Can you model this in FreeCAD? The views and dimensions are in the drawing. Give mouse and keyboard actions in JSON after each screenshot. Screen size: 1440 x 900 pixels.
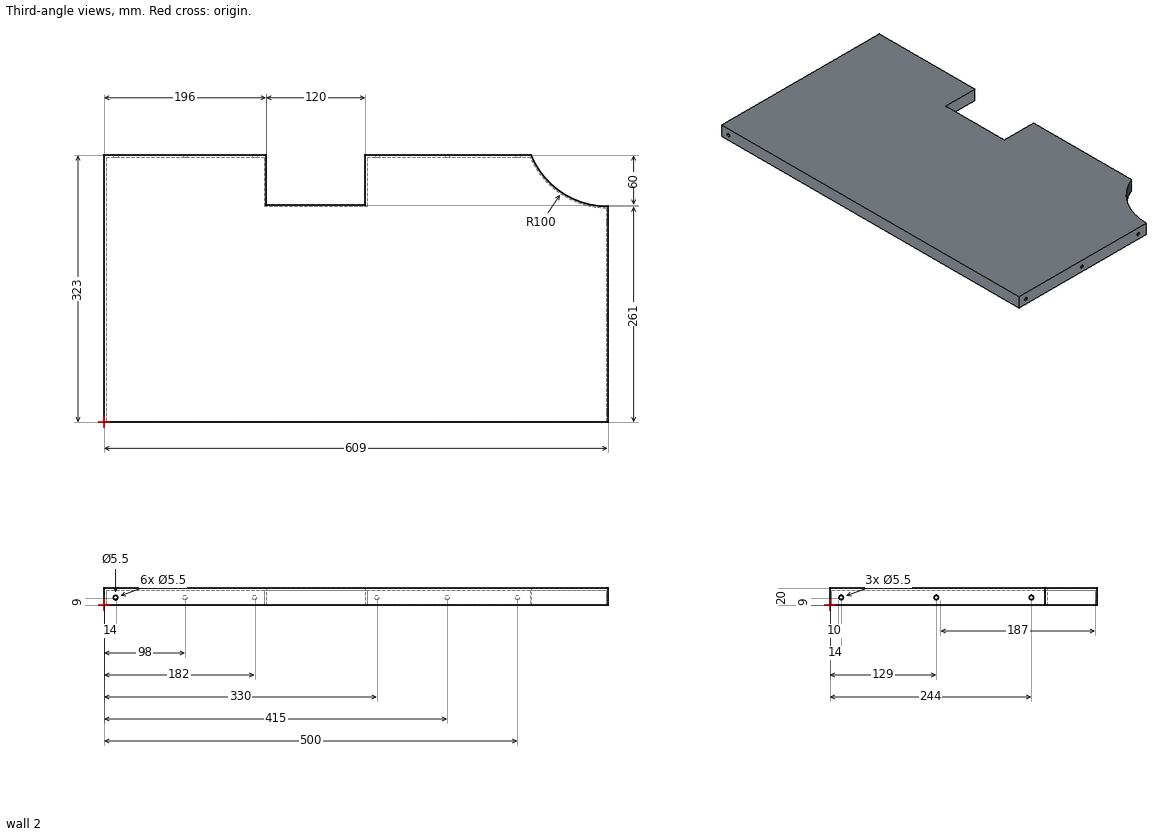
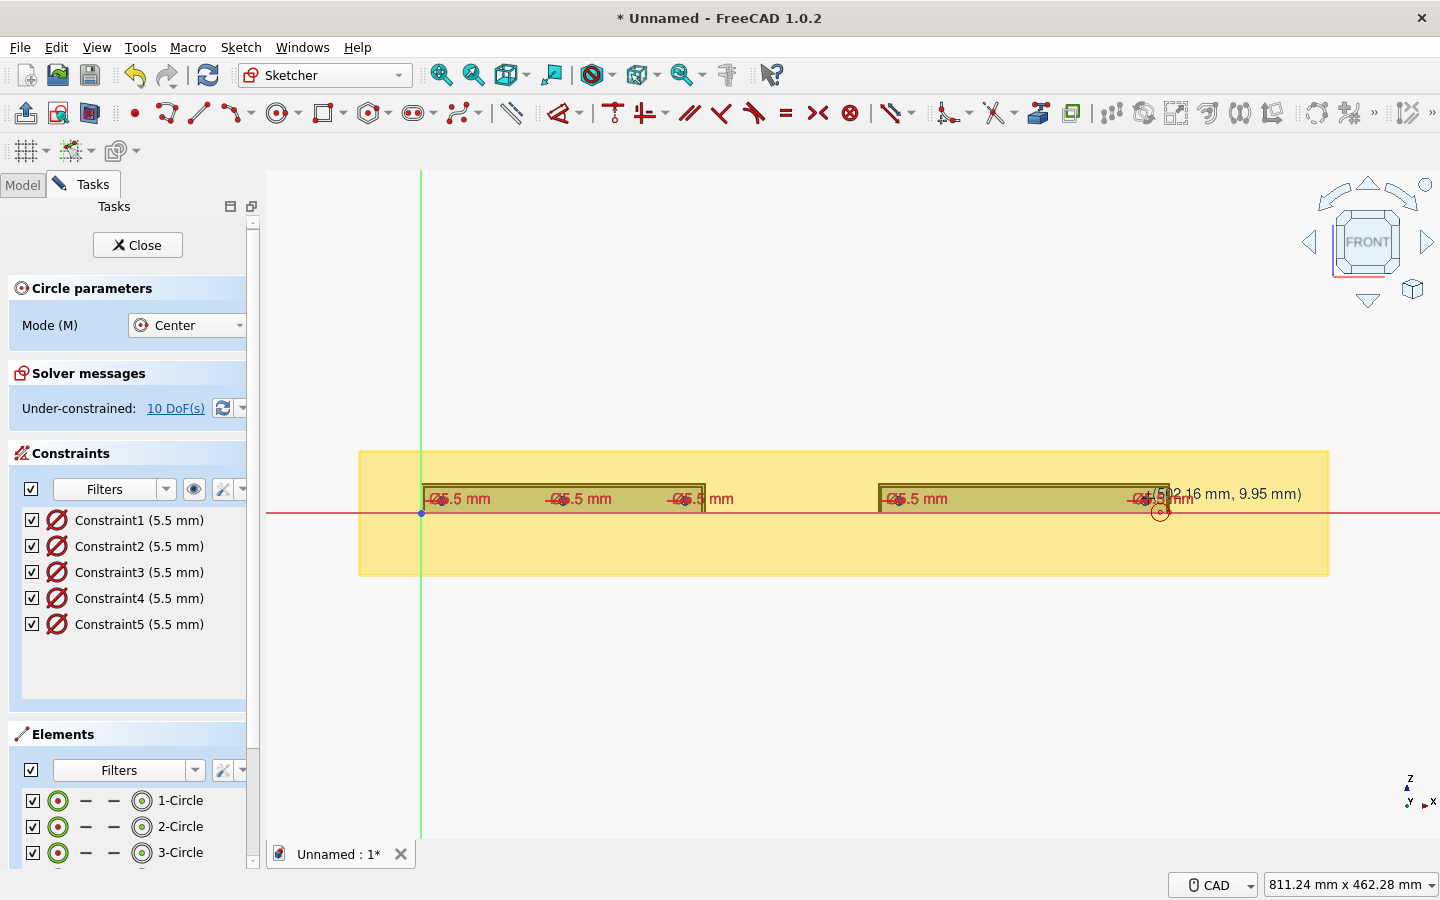
{"action": "scroll", "coordinate": [1022, 500], "scroll_direction": "up", "scroll_amount": 9}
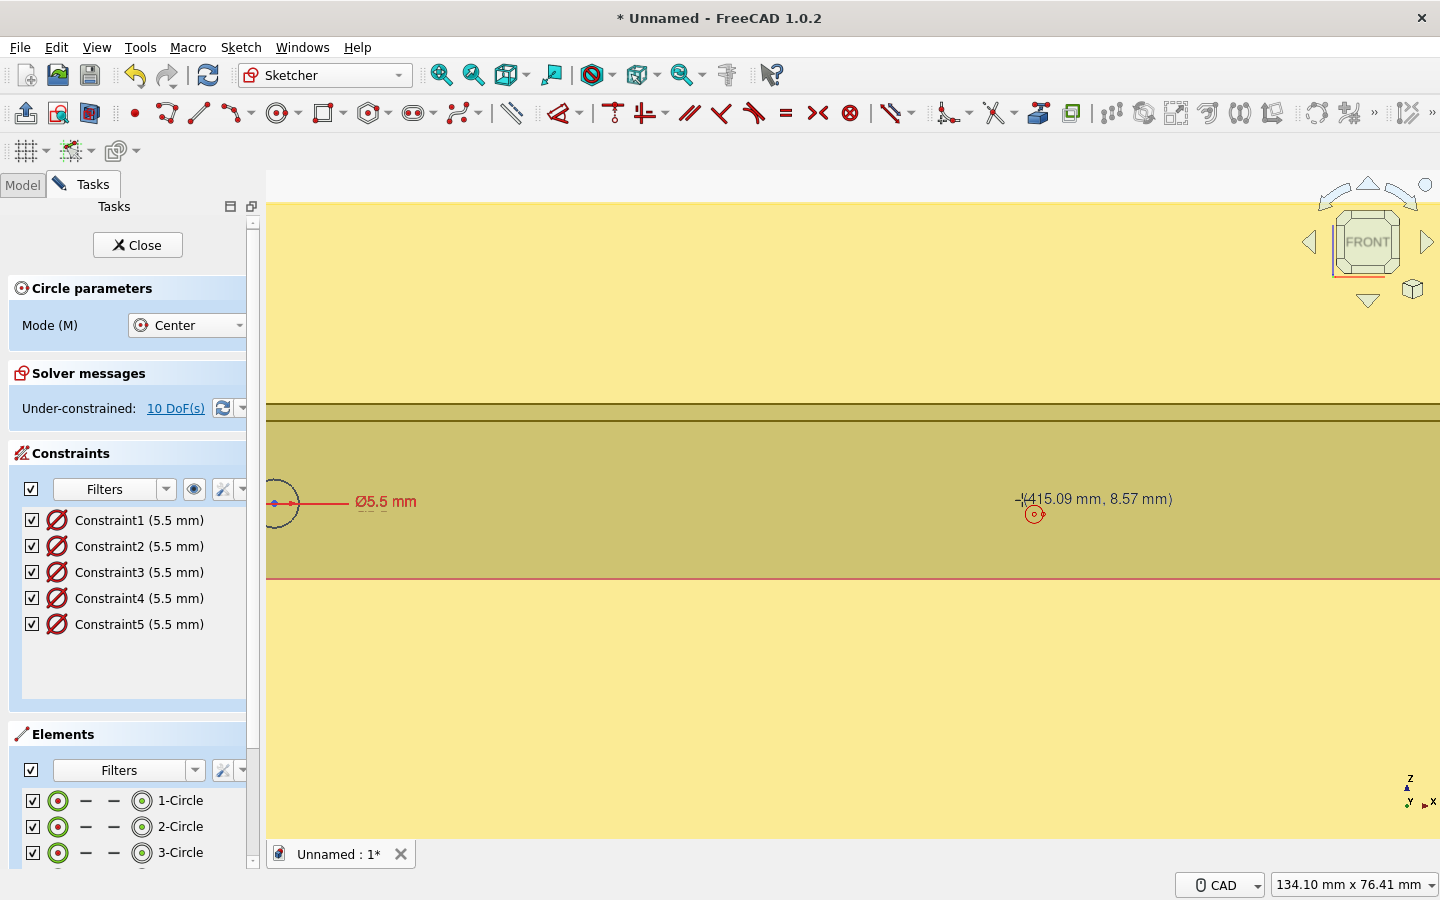
{"action": "scroll", "coordinate": [1022, 500], "scroll_direction": "down", "scroll_amount": 9}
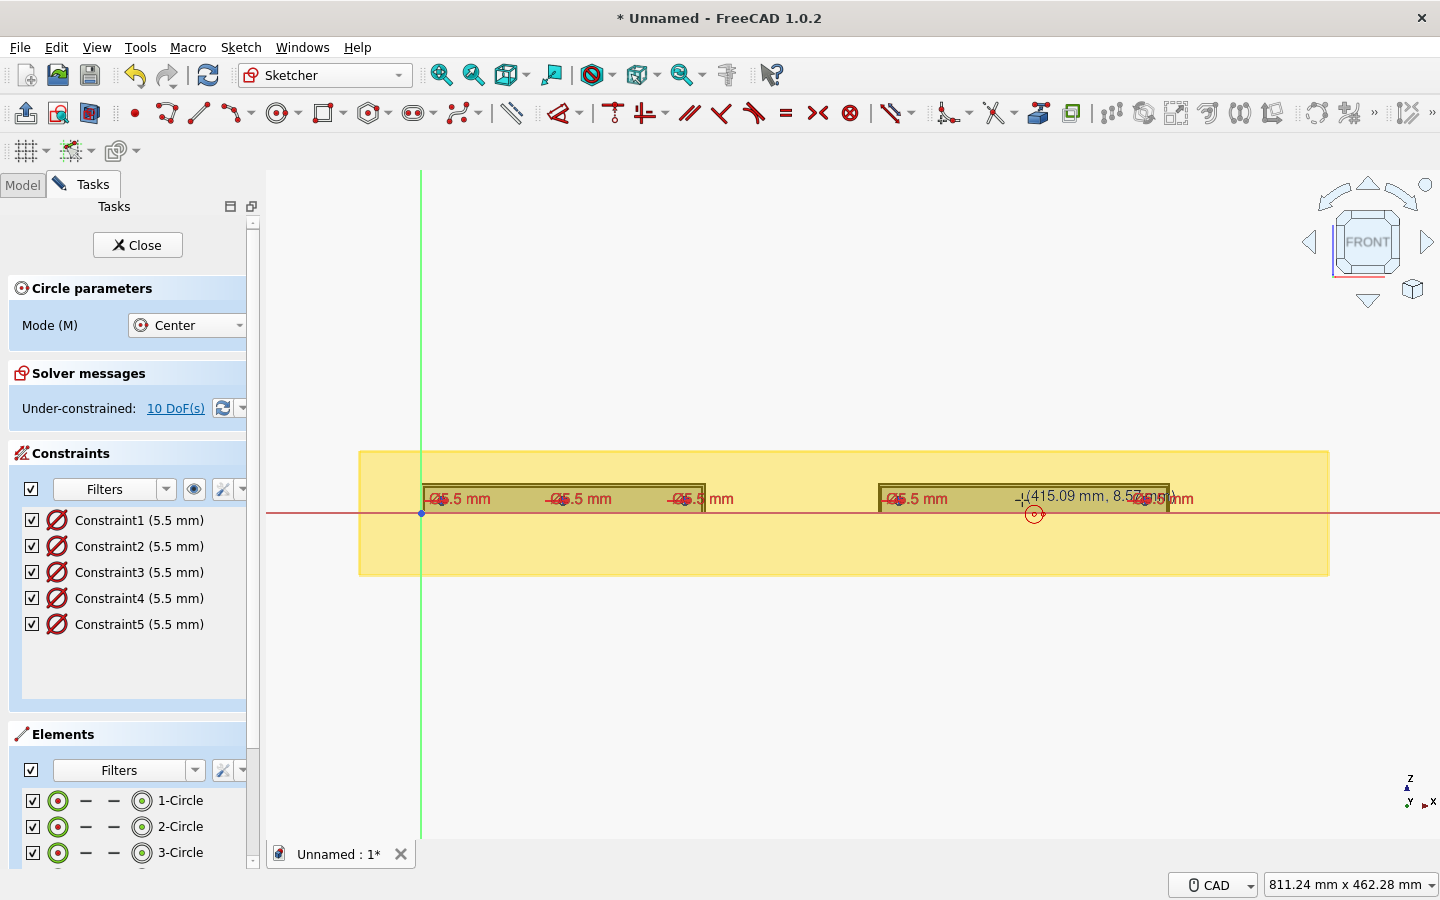
{"action": "left_click", "coordinate": [1022, 500]}
{"action": "mouse_move", "coordinate": [1025, 498]}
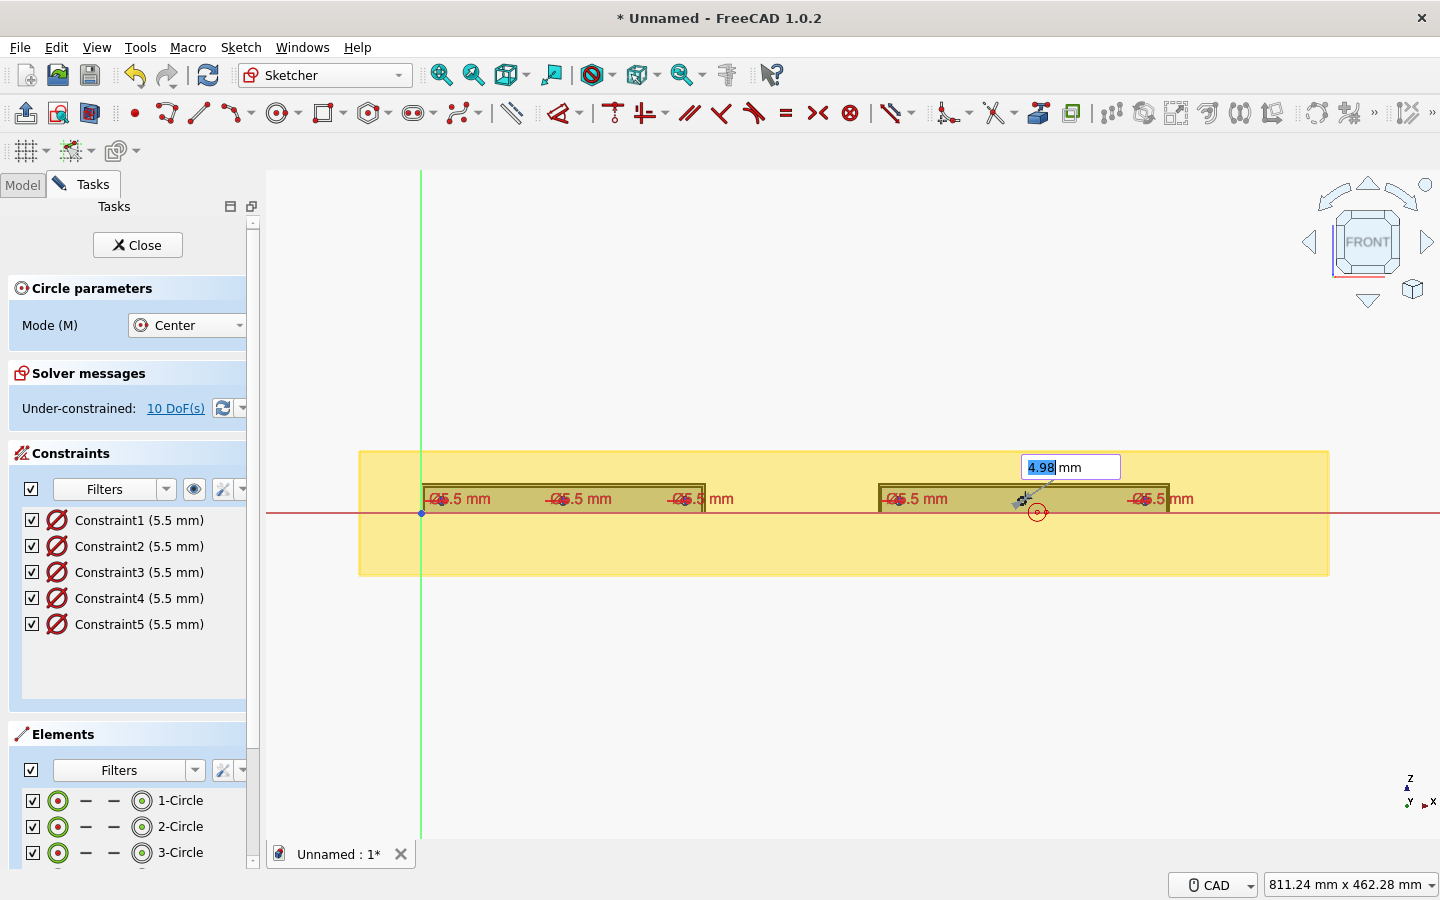
{"action": "type", "text": "5.5"}
{"action": "key", "text": "Return"}
{"action": "key", "text": "Escape"}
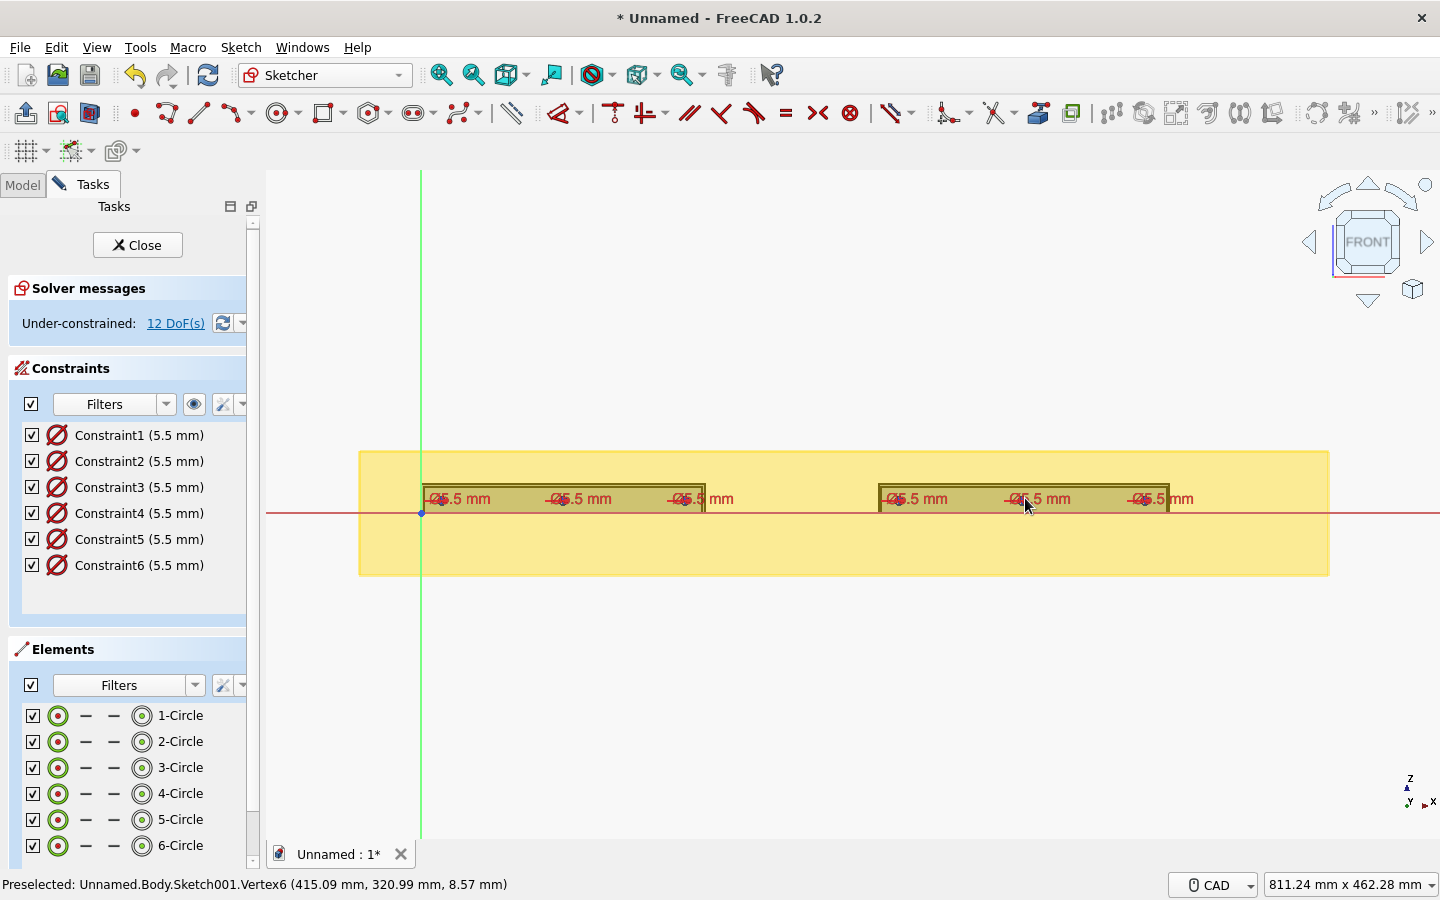
{"action": "key", "text": "d"}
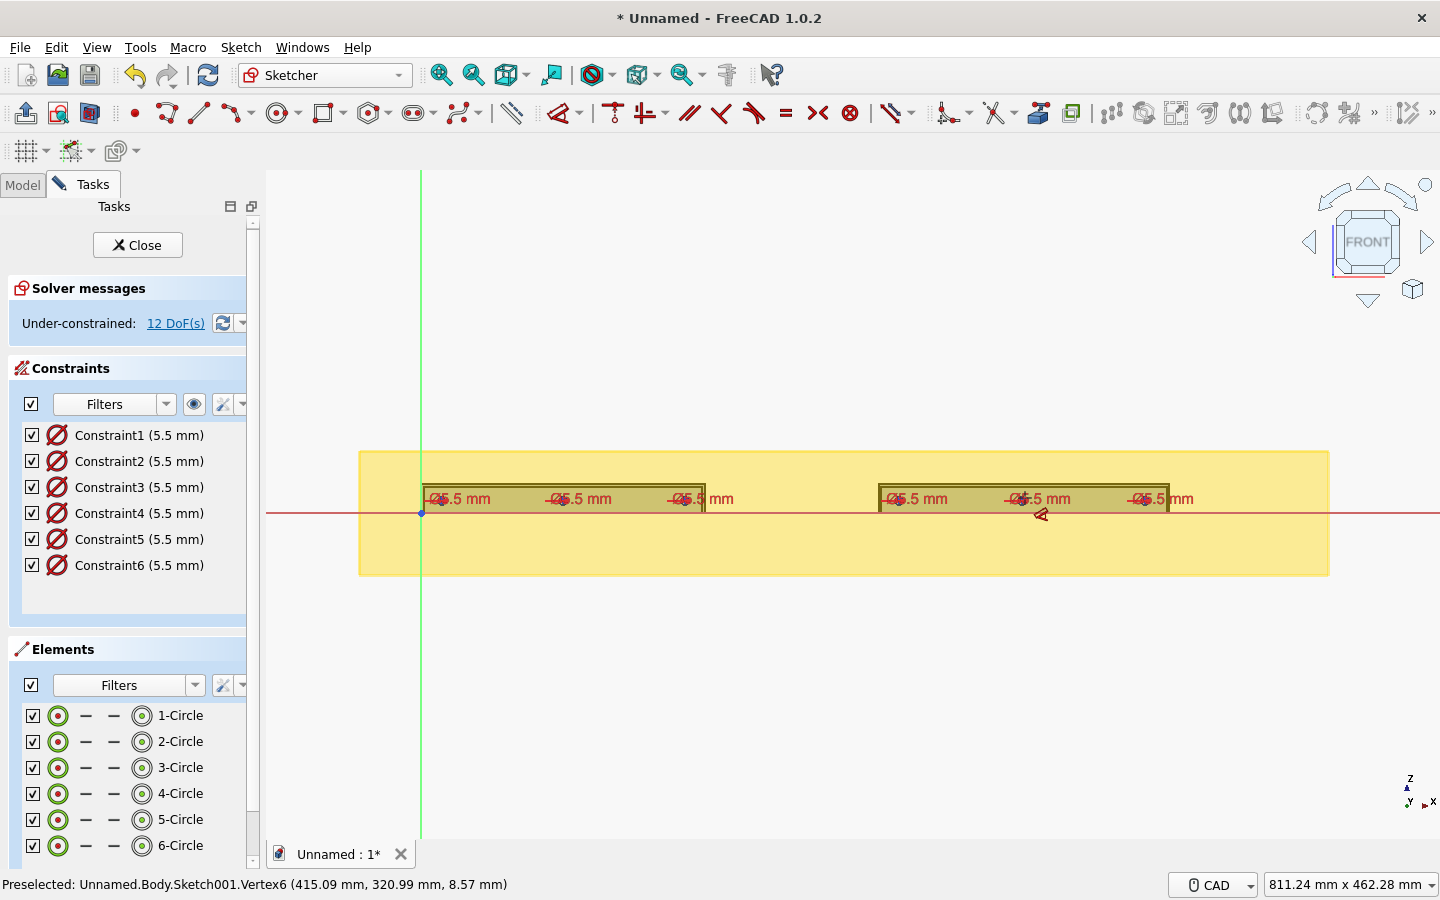
{"action": "scroll", "coordinate": [442, 501], "scroll_direction": "up", "scroll_amount": 6}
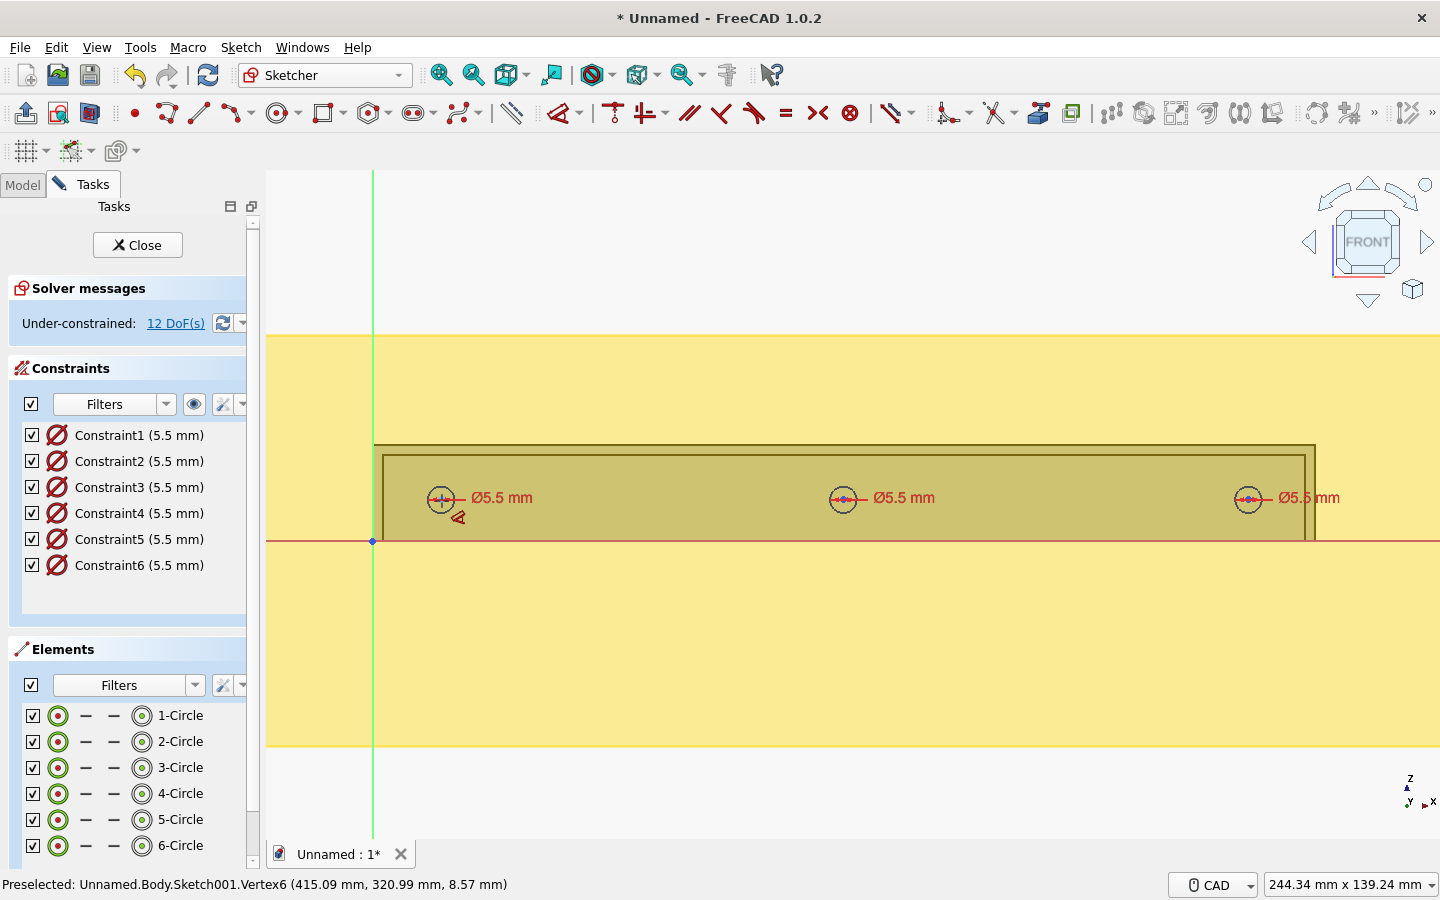
{"action": "left_click", "coordinate": [441, 500]}
{"action": "left_click", "coordinate": [339, 520]}